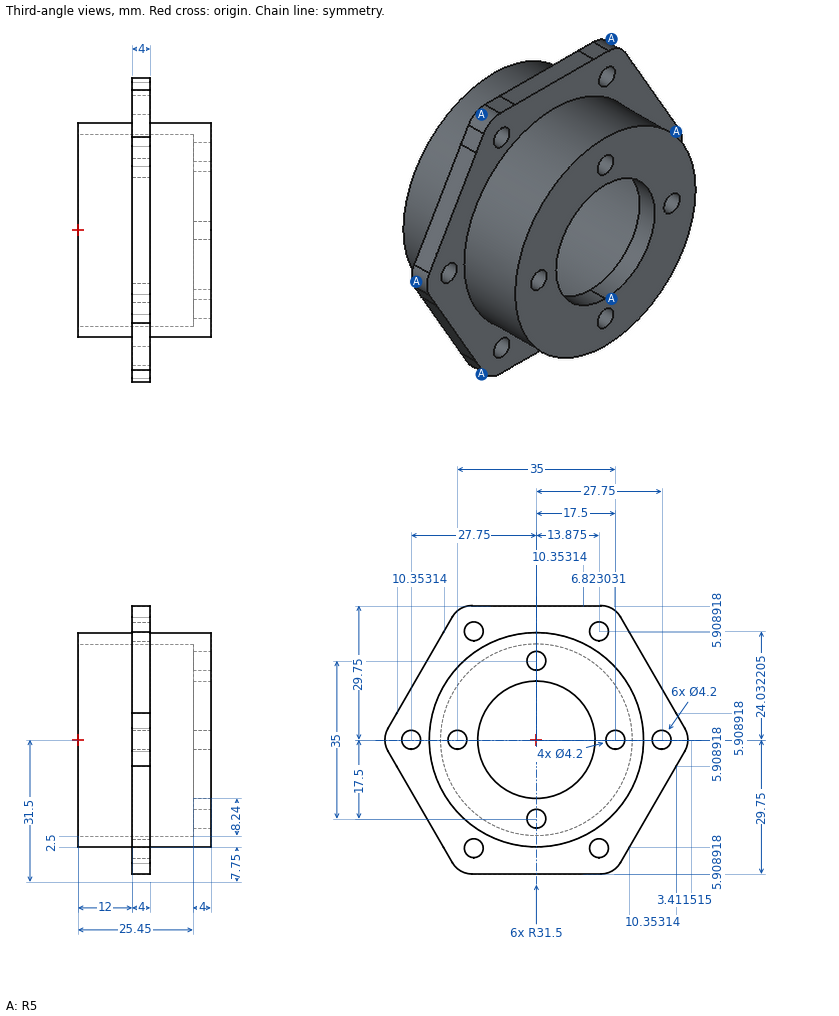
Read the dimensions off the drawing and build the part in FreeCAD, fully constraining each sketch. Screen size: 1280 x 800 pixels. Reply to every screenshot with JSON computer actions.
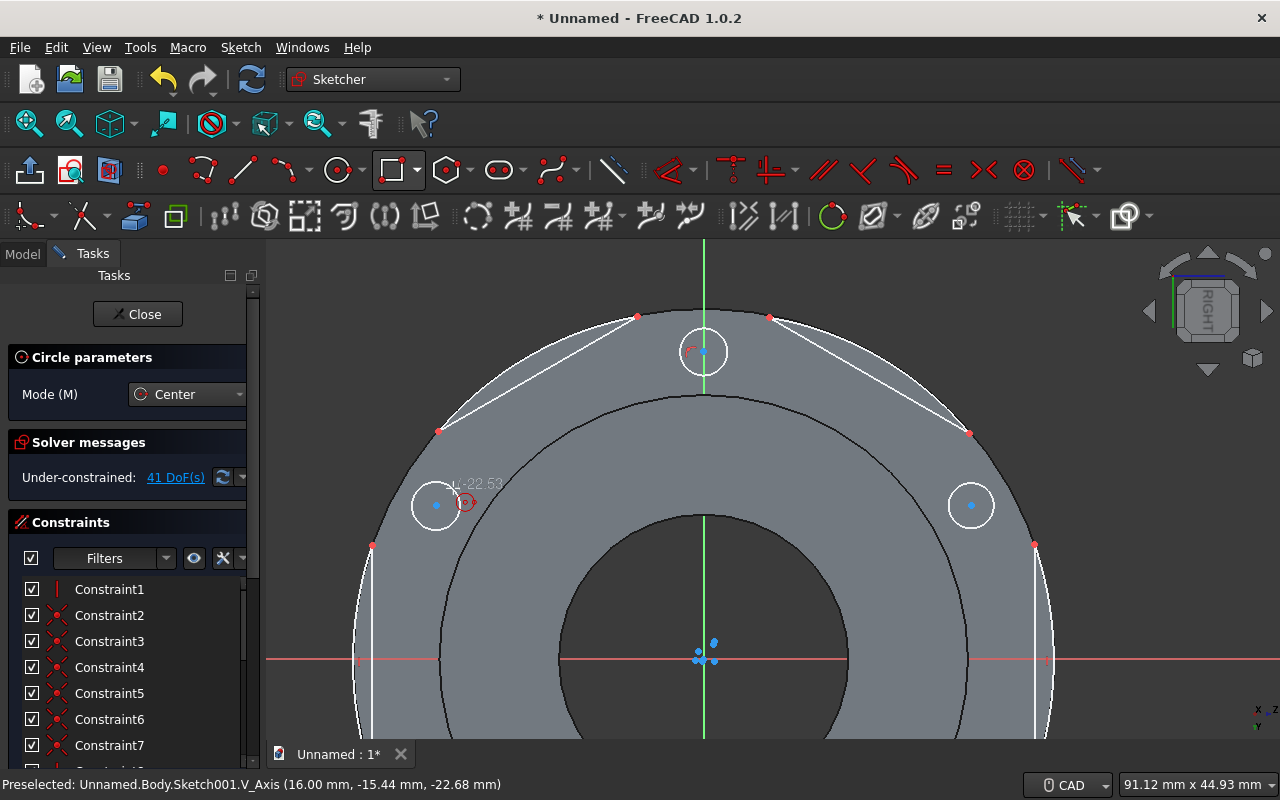
{"action": "scroll", "coordinate": [705, 350], "scroll_direction": "down", "scroll_amount": 4}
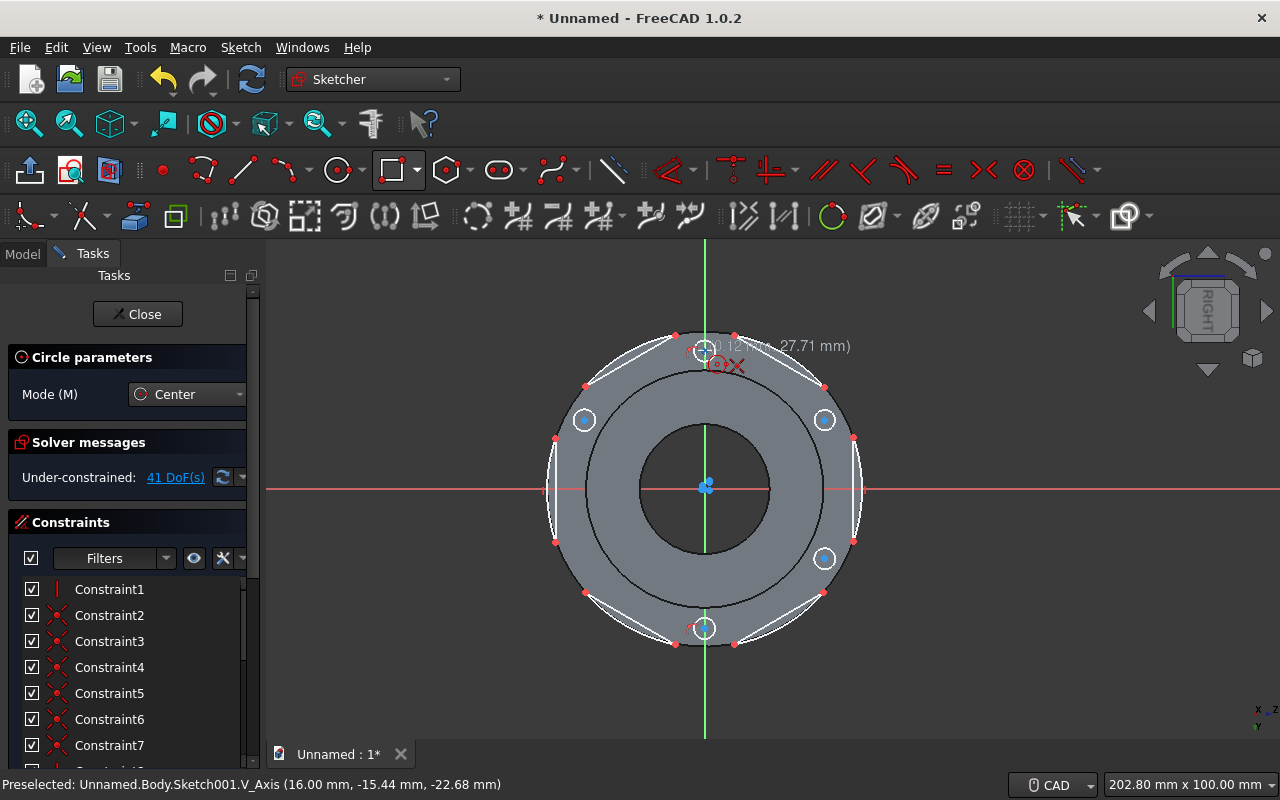
{"action": "scroll", "coordinate": [584, 558], "scroll_direction": "up", "scroll_amount": 4}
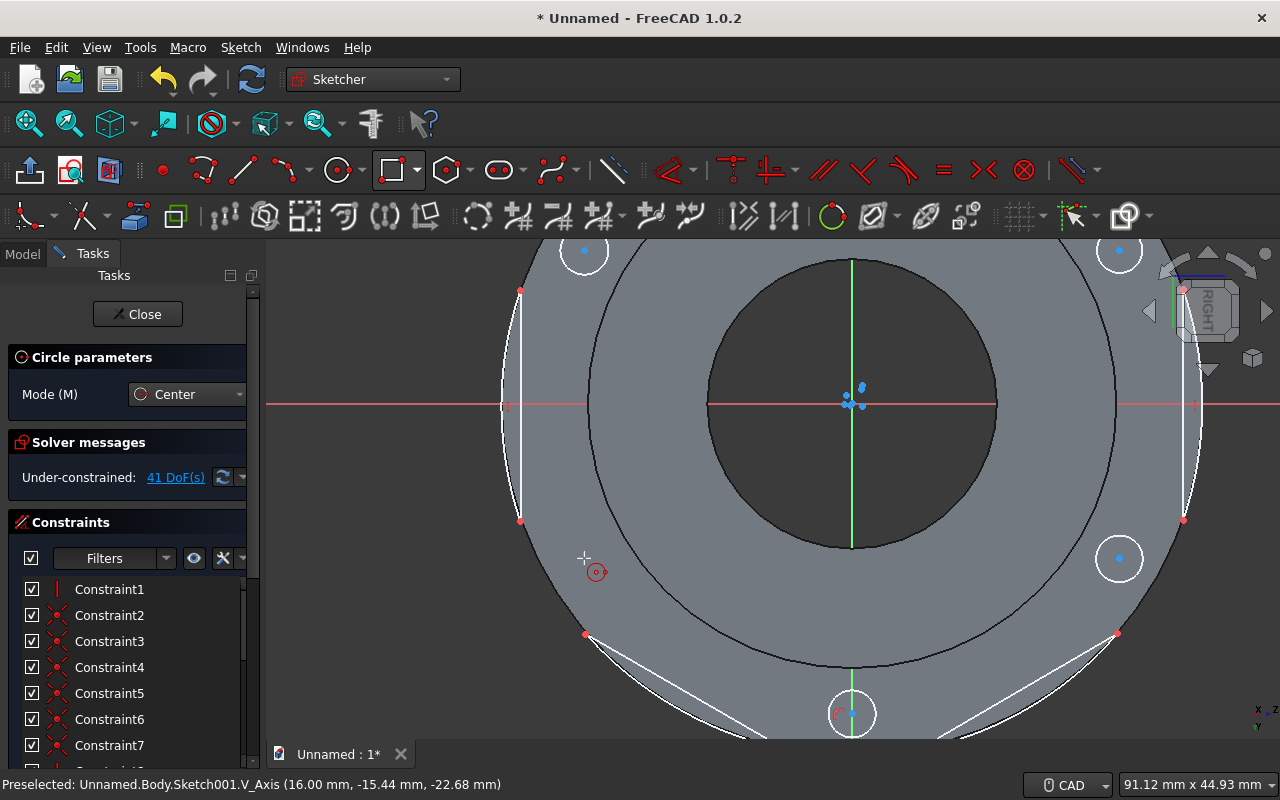
{"action": "left_click", "coordinate": [585, 558]}
{"action": "left_click", "coordinate": [601, 542]}
{"action": "key", "text": "Escape"}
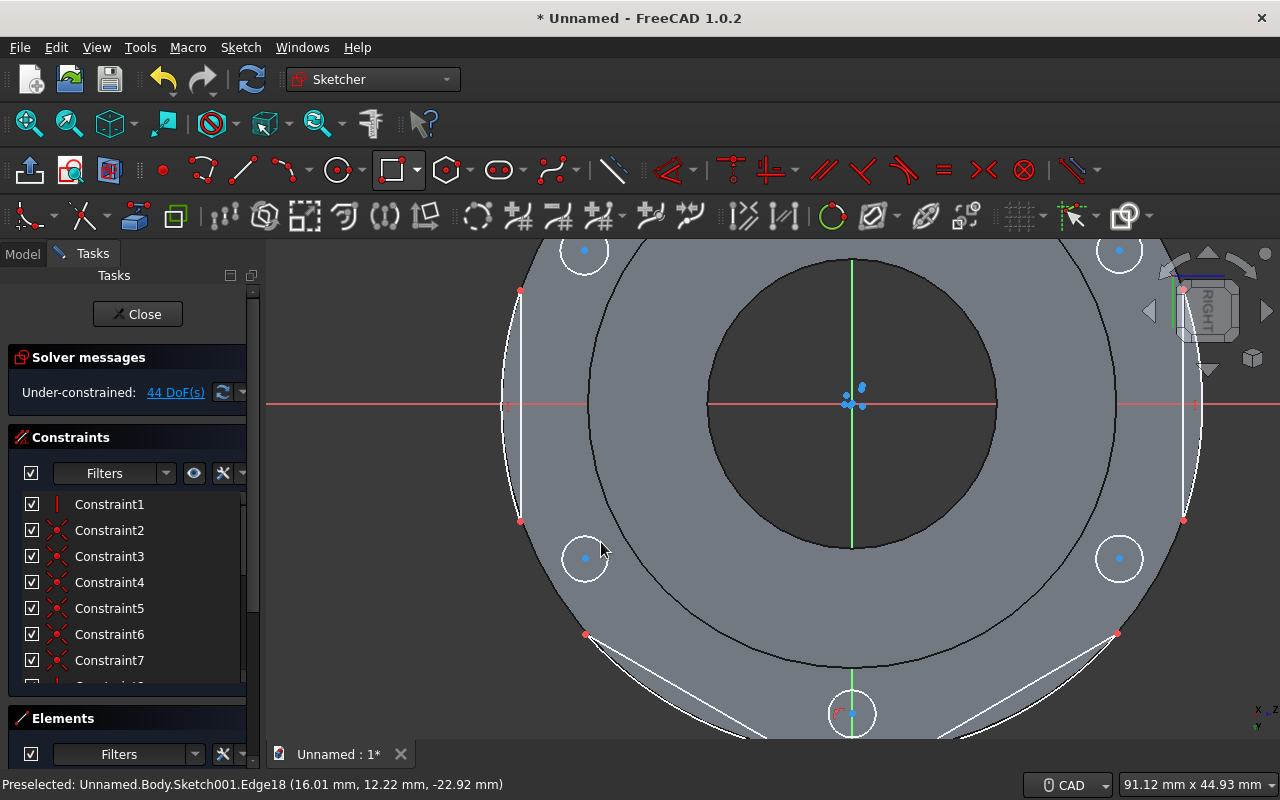
{"action": "left_click", "coordinate": [505, 359]}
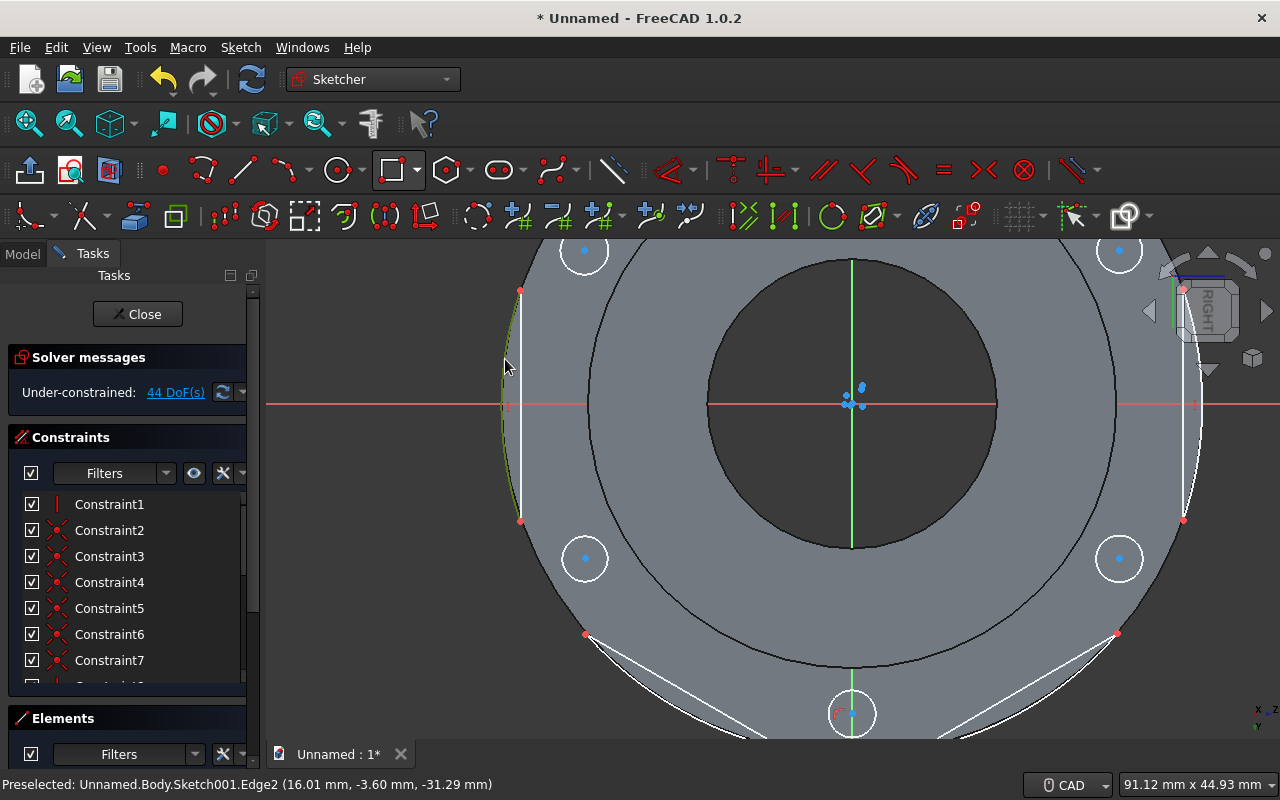
{"action": "left_click", "coordinate": [638, 682]}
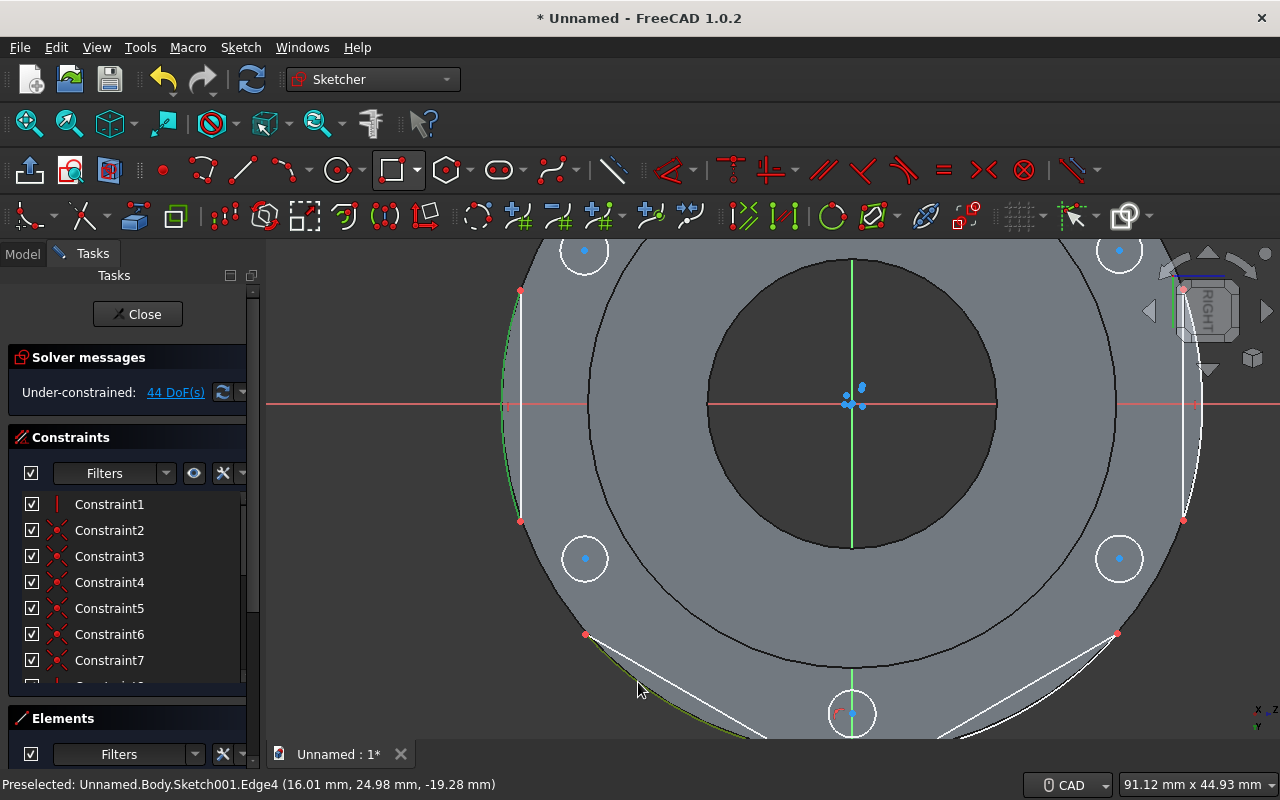
{"action": "key", "text": "c"}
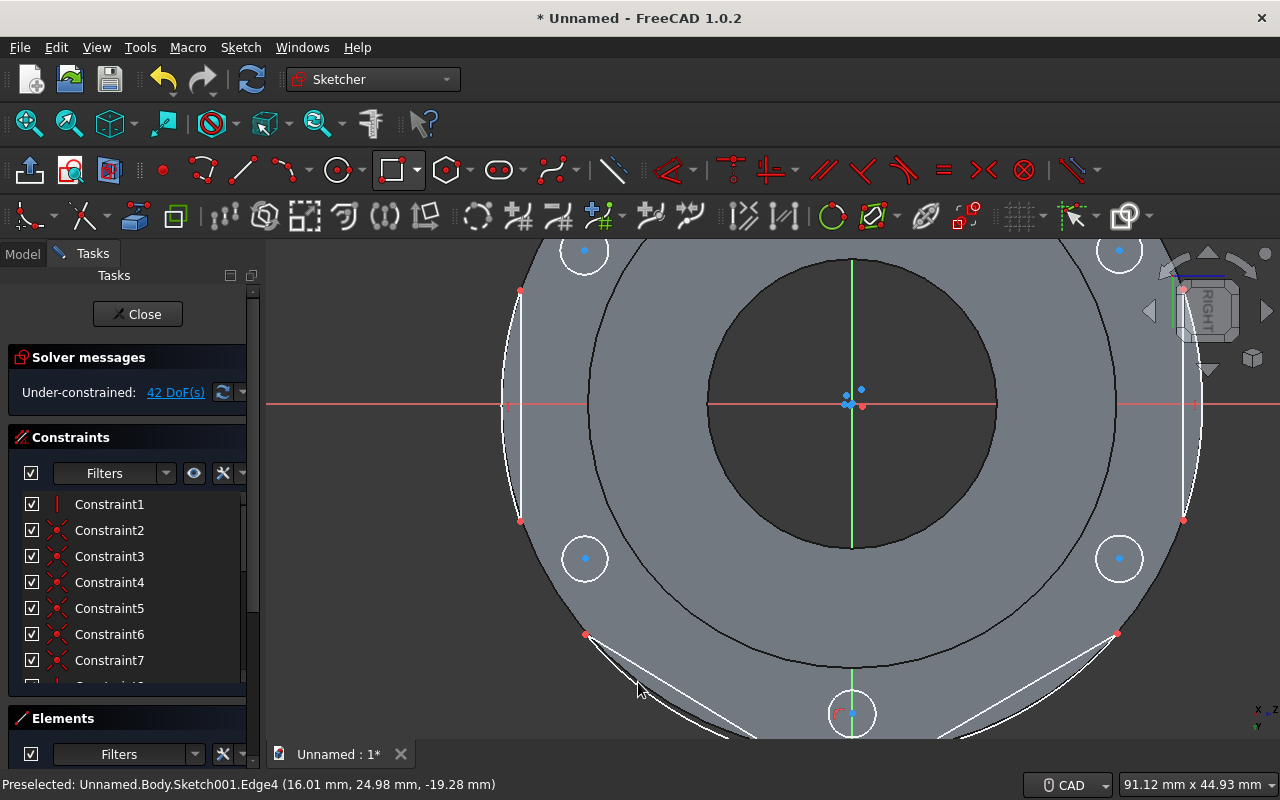
{"action": "left_click", "coordinate": [505, 359]}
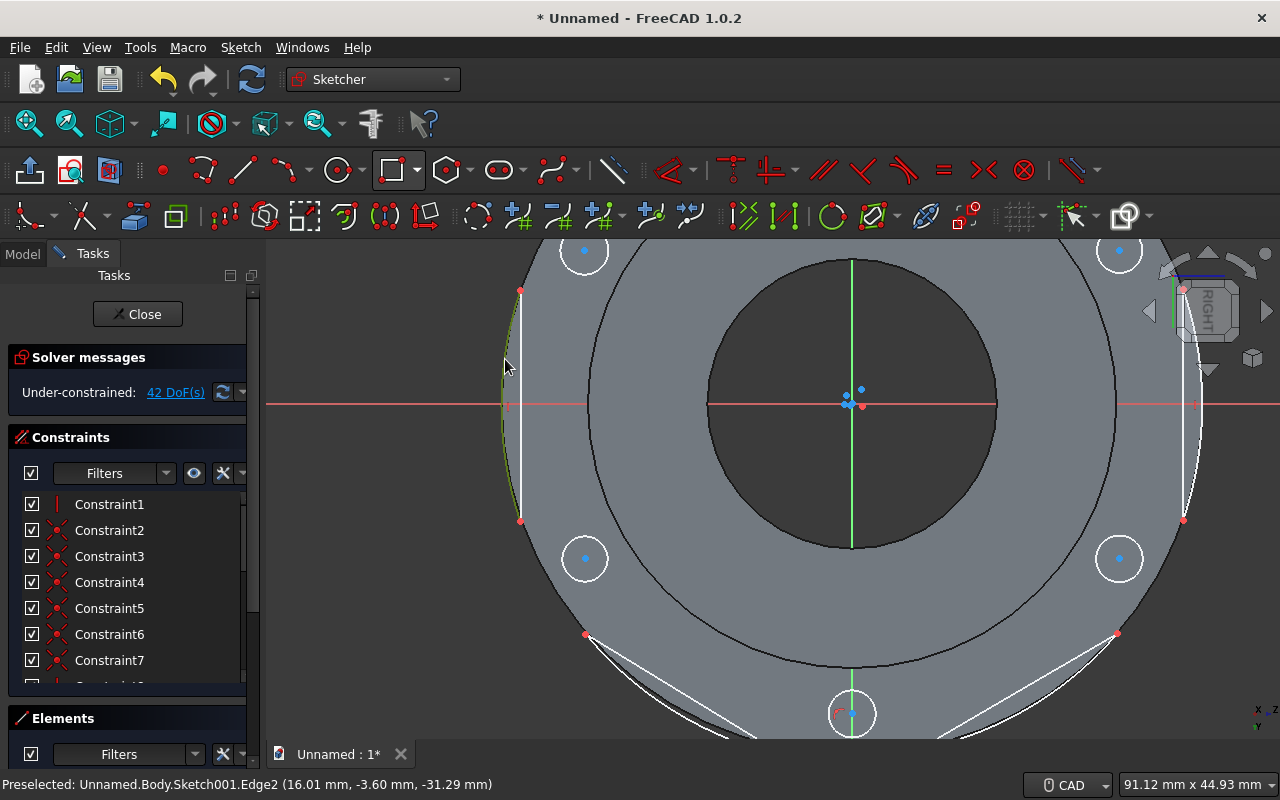
{"action": "left_click", "coordinate": [1066, 682]}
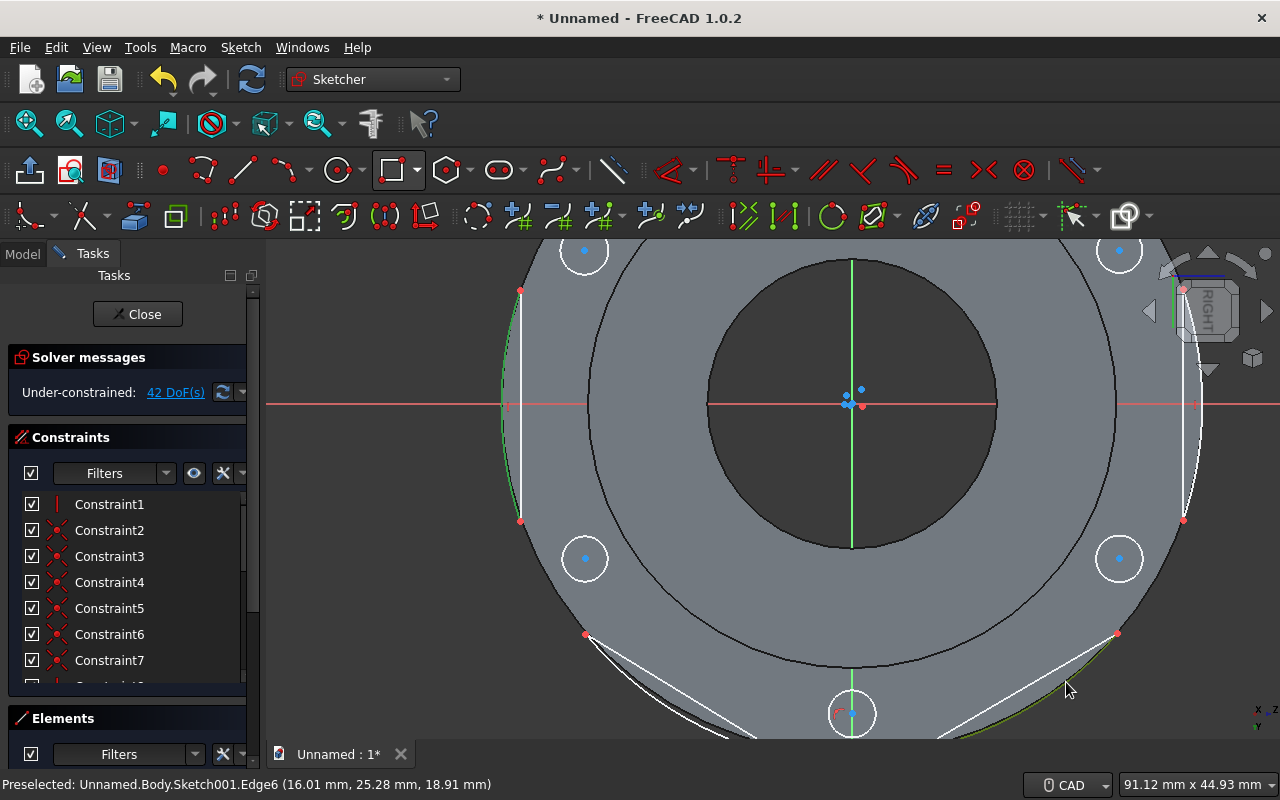
{"action": "left_click", "coordinate": [732, 170]}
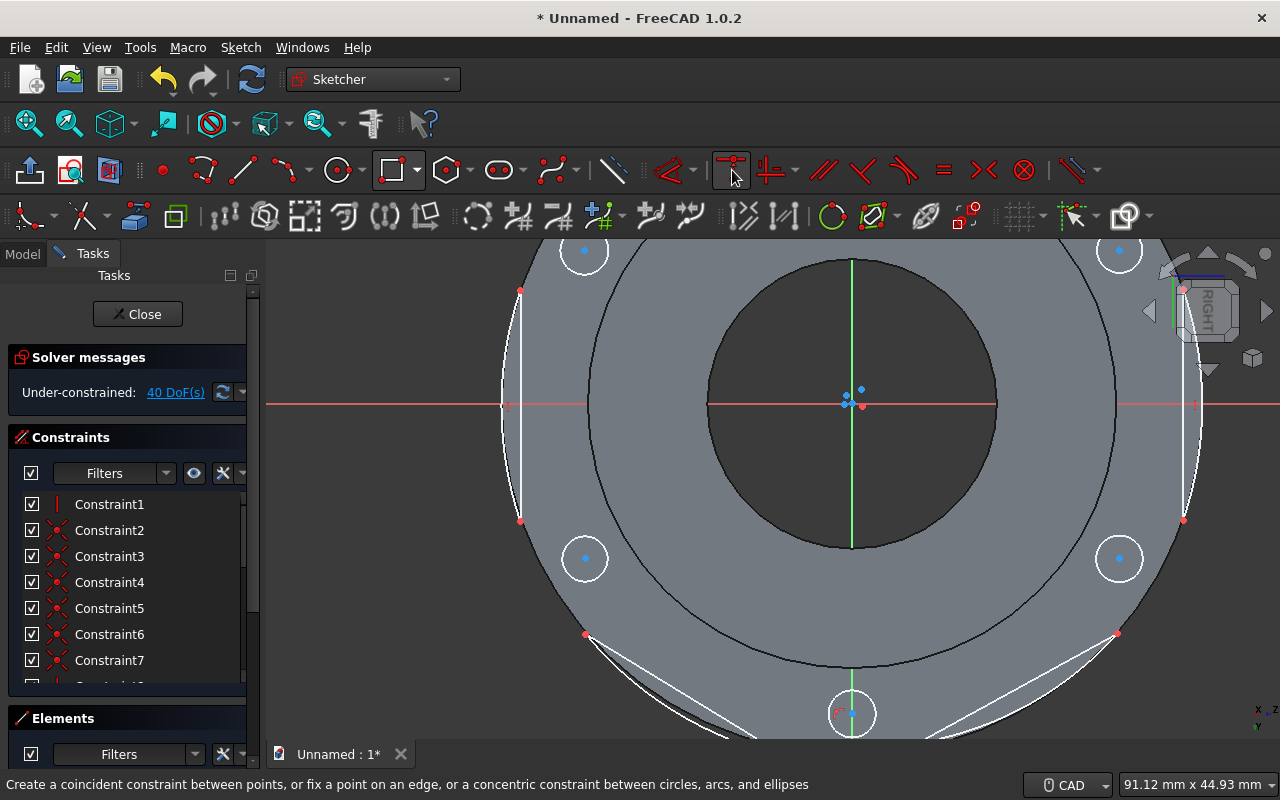
{"action": "left_click", "coordinate": [505, 359]}